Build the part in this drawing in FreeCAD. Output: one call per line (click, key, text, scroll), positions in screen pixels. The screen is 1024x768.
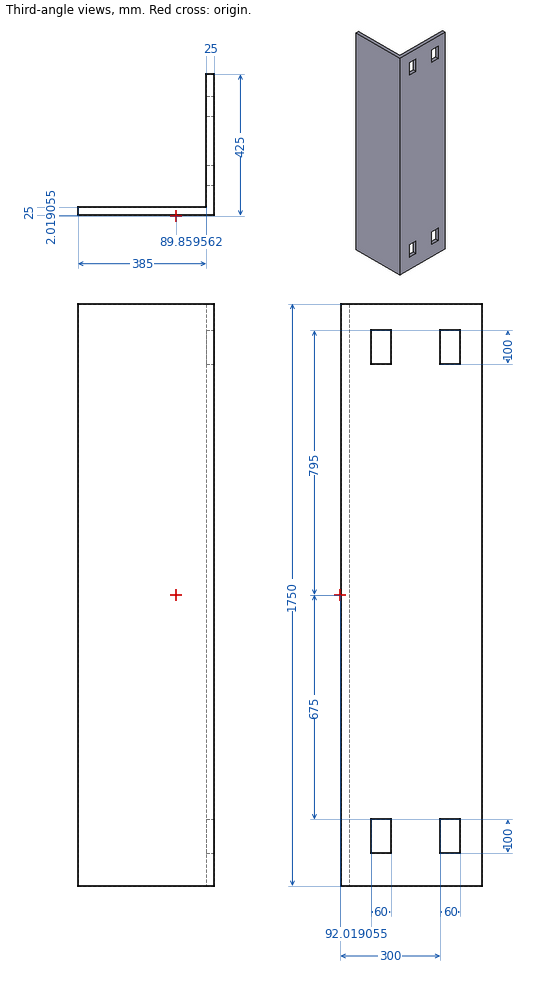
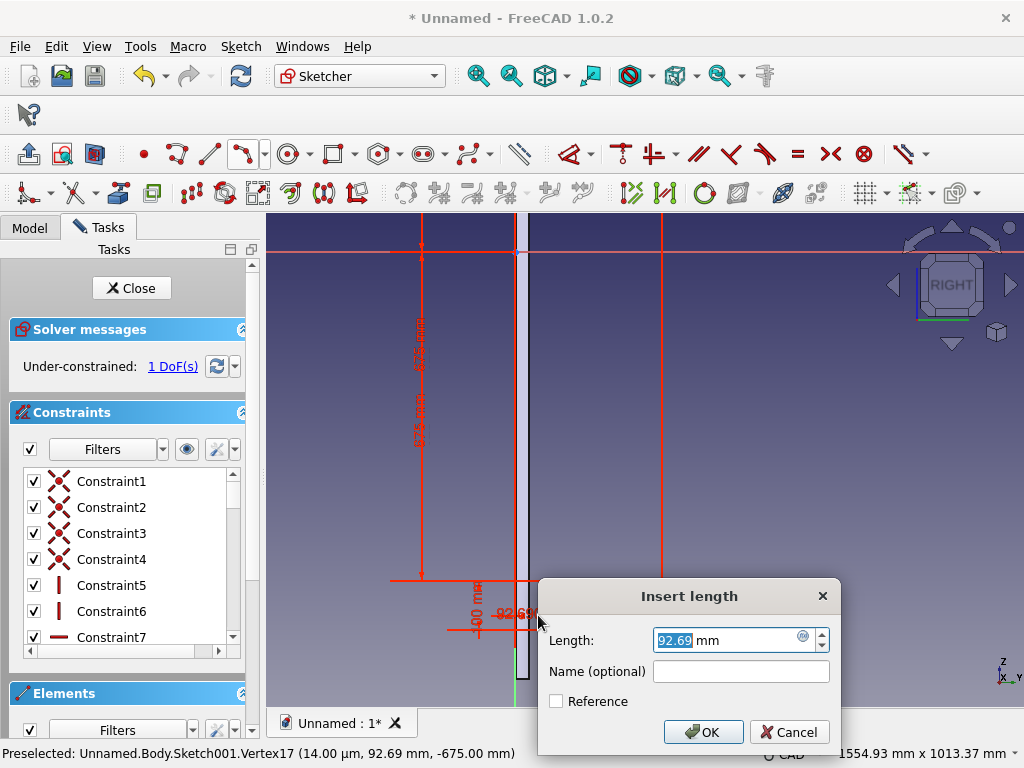
text(92.019055)
key(Return)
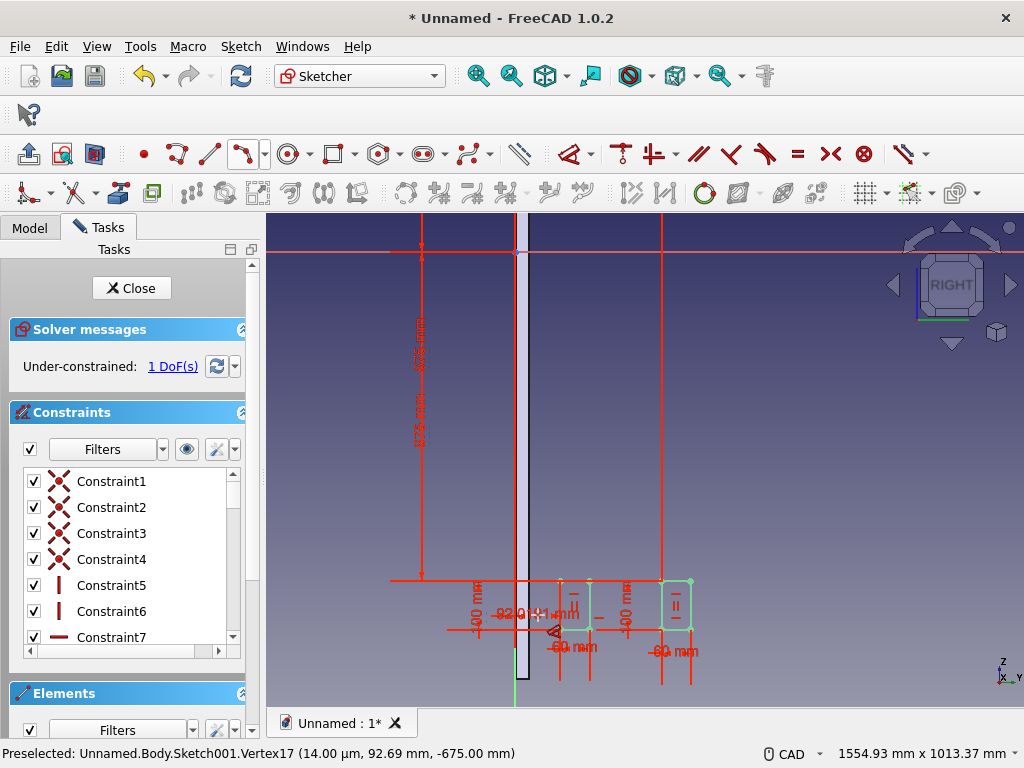
scroll(561, 584, down, 5)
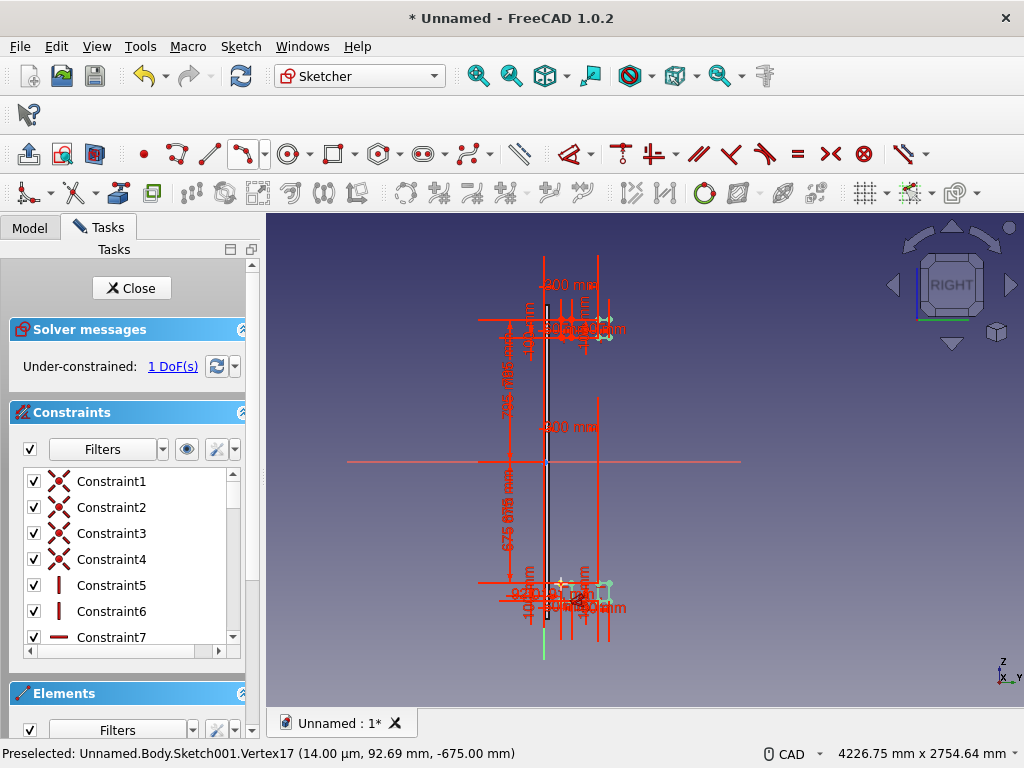
scroll(561, 320, up, 5)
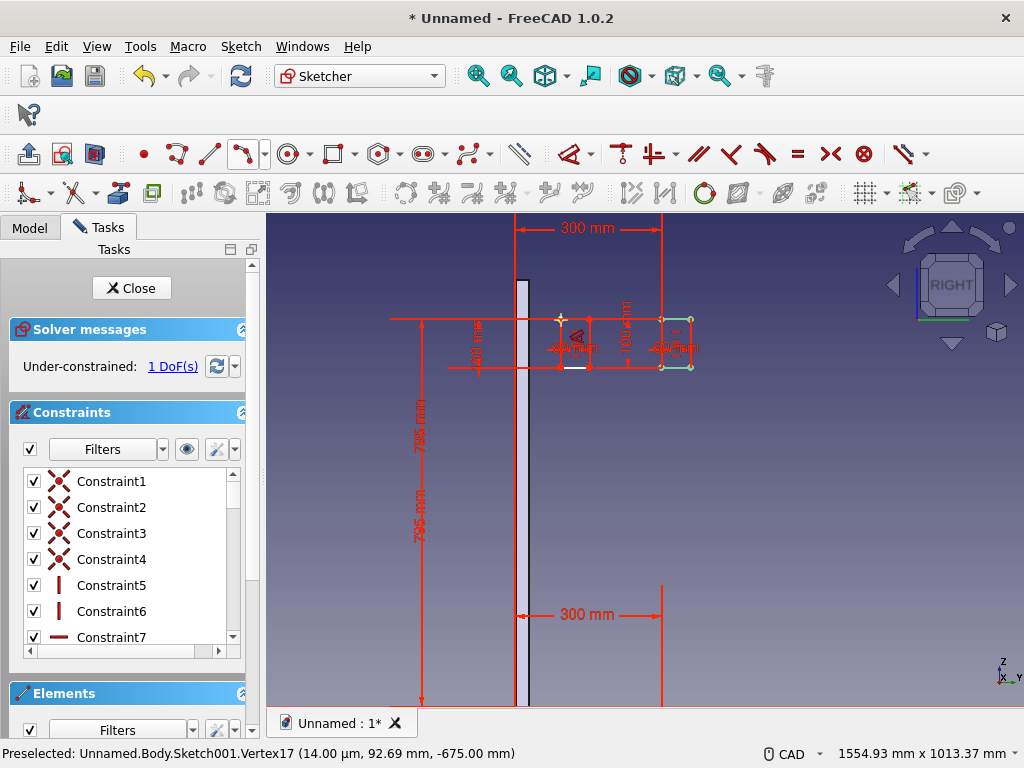
click(561, 319)
click(538, 285)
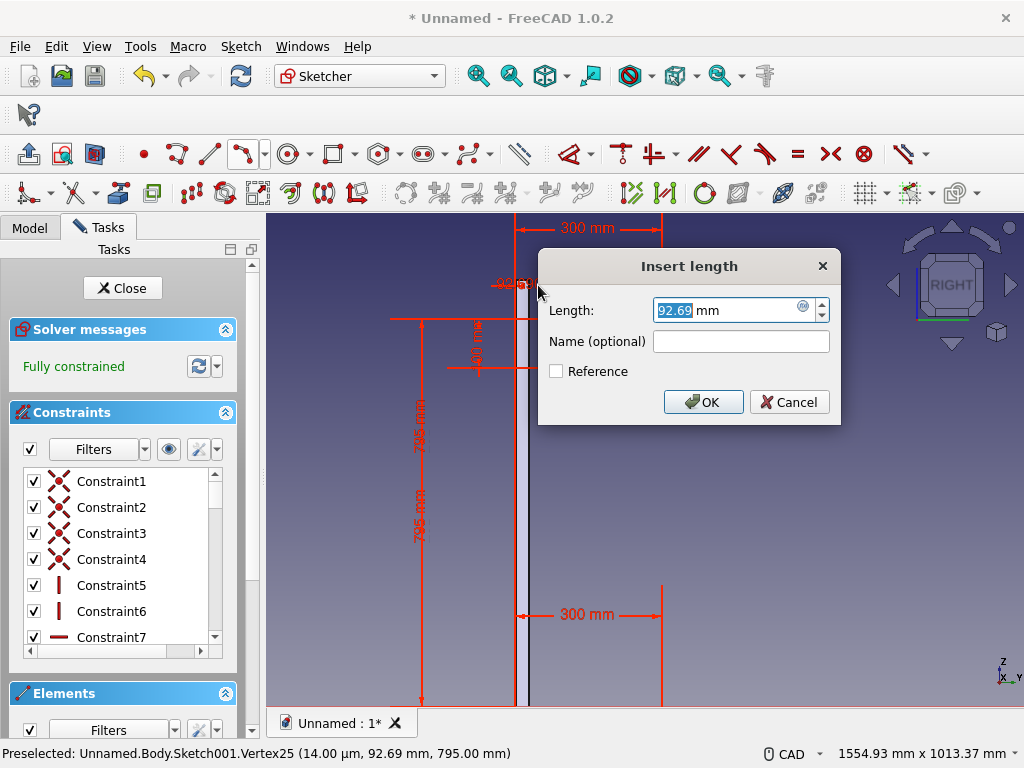
text(92.019055)
key(Return)
key(Escape)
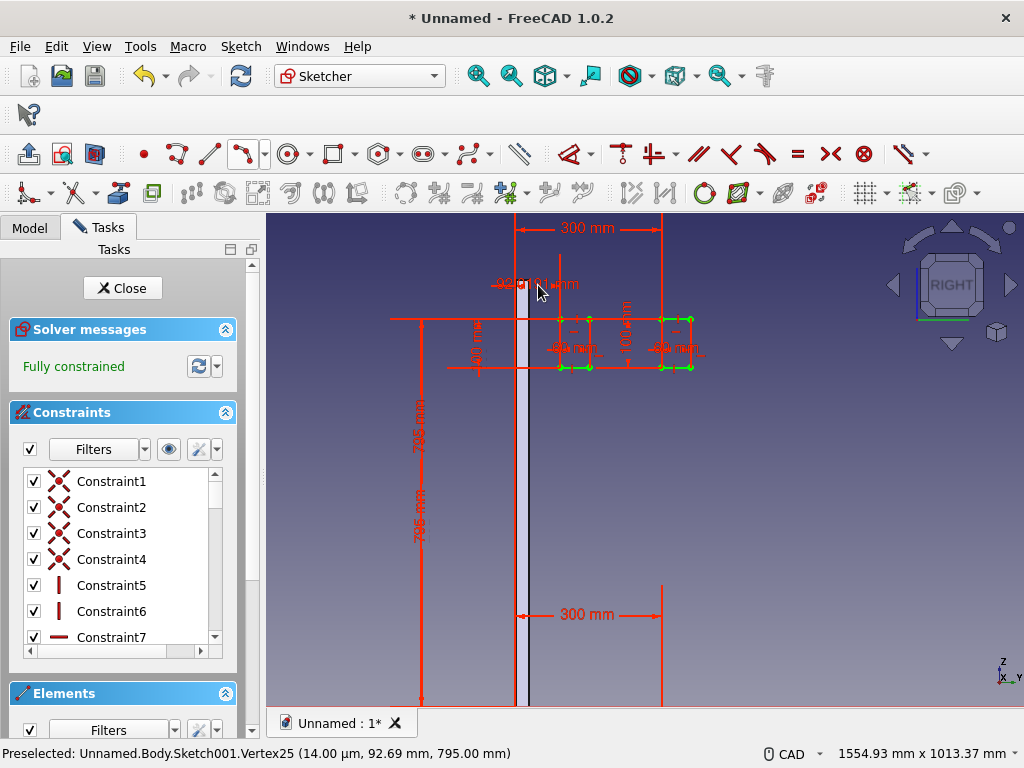
click(123, 288)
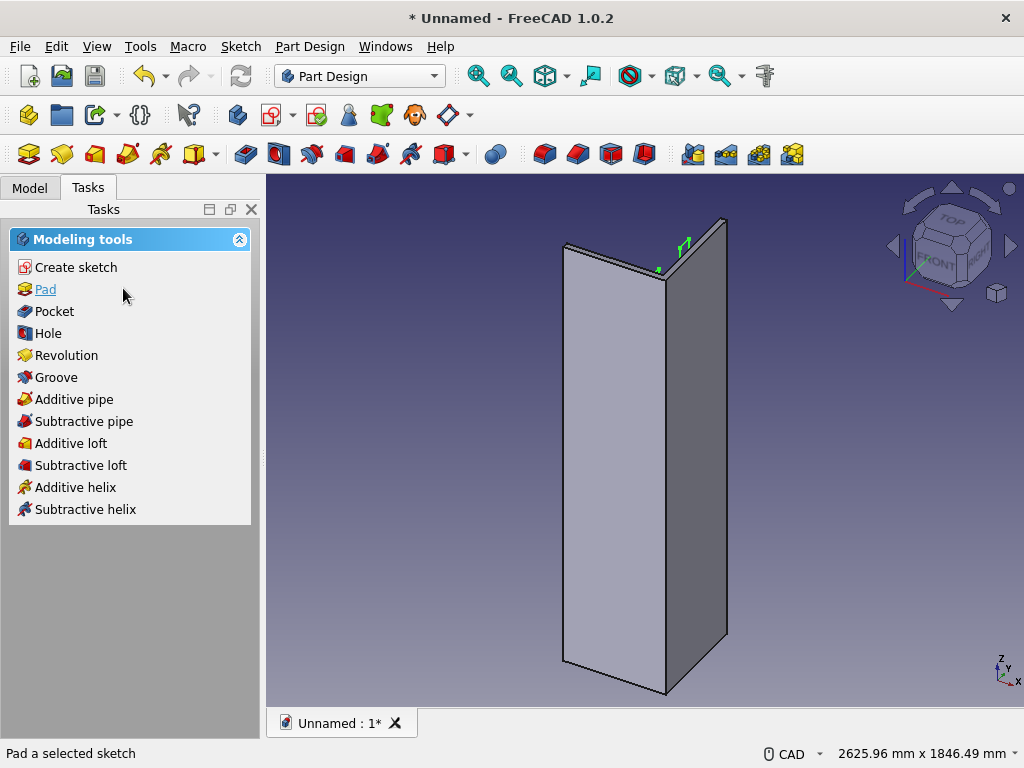
click(246, 154)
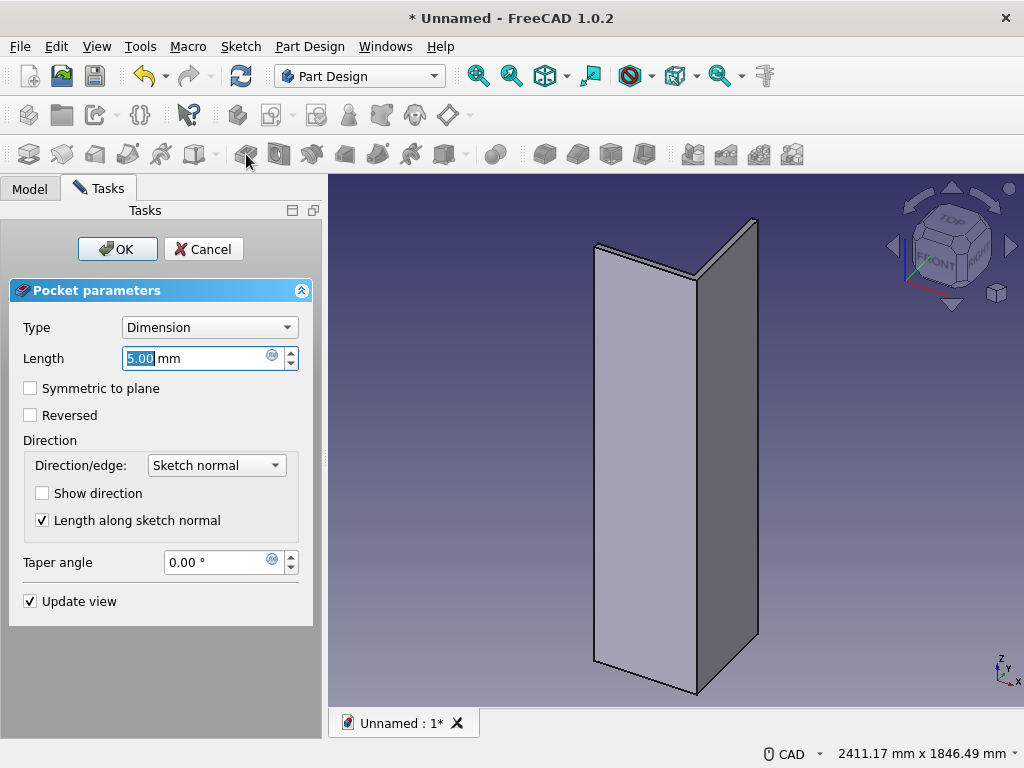
click(210, 328)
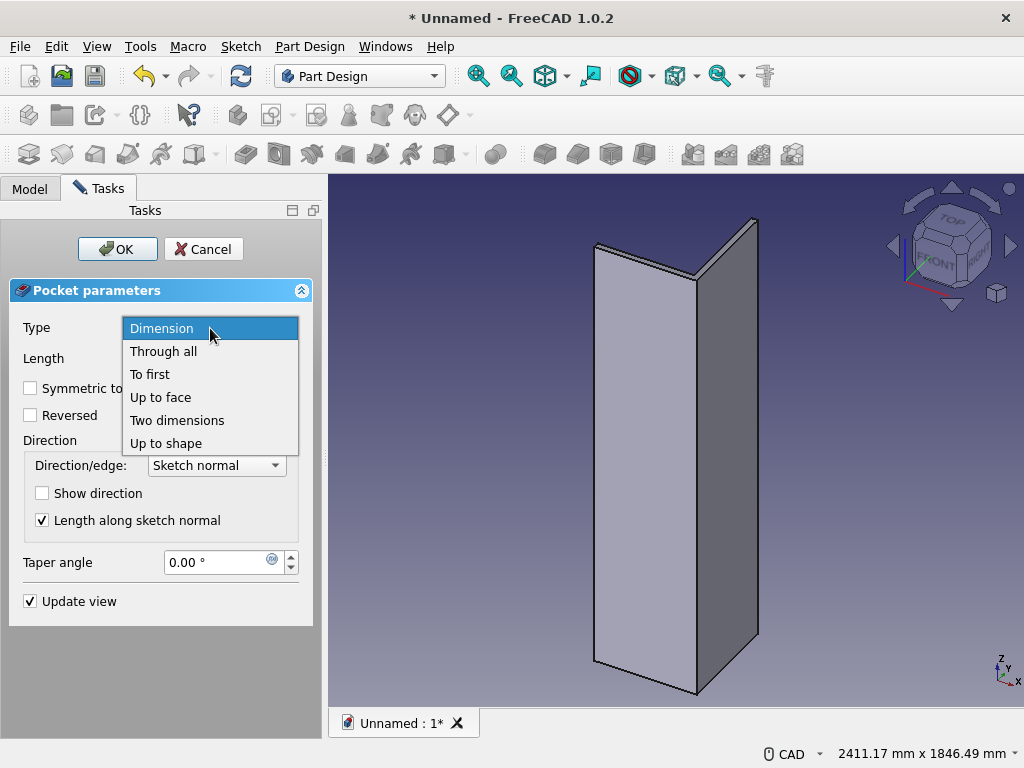
click(208, 352)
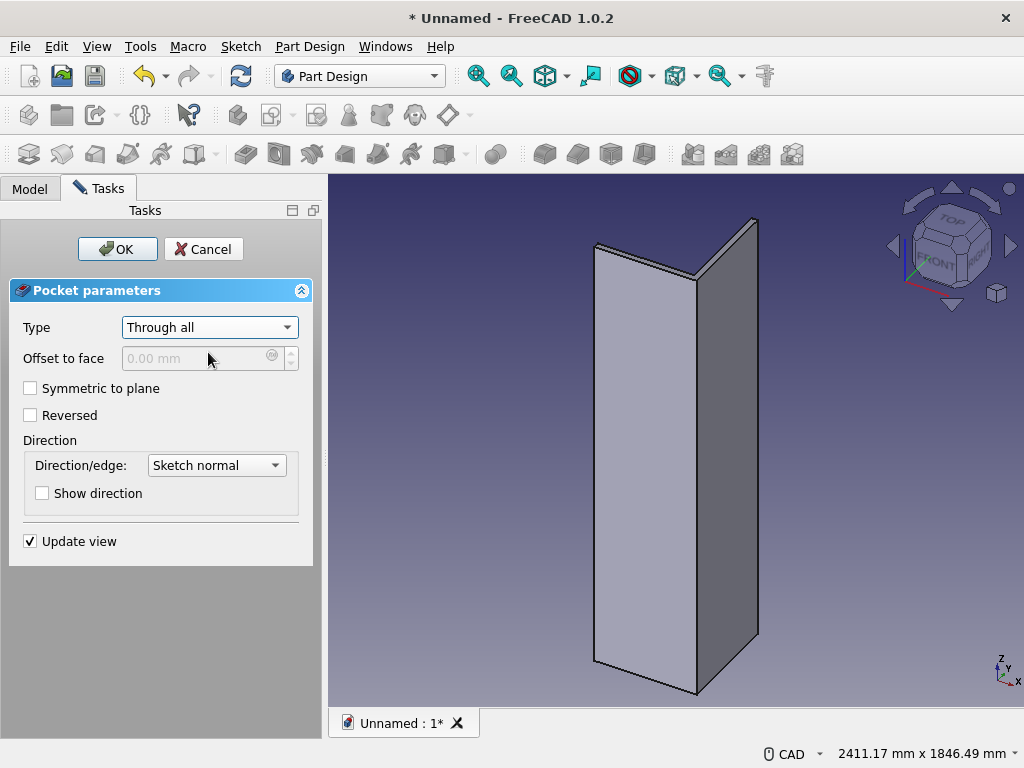
click(31, 415)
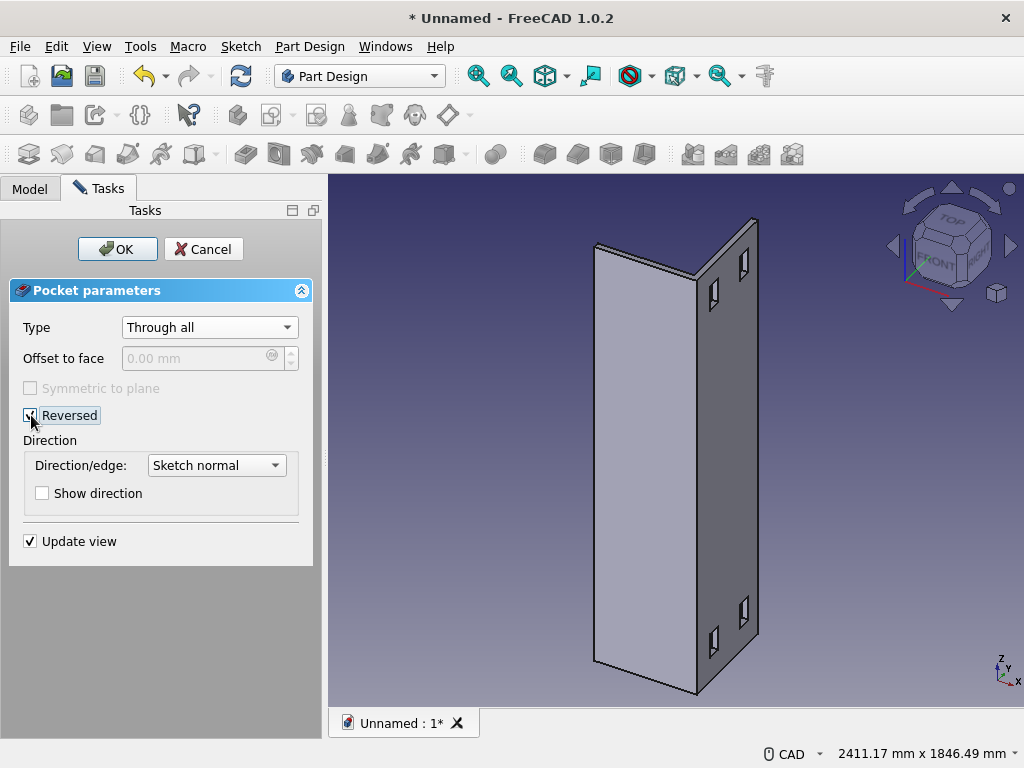
click(118, 249)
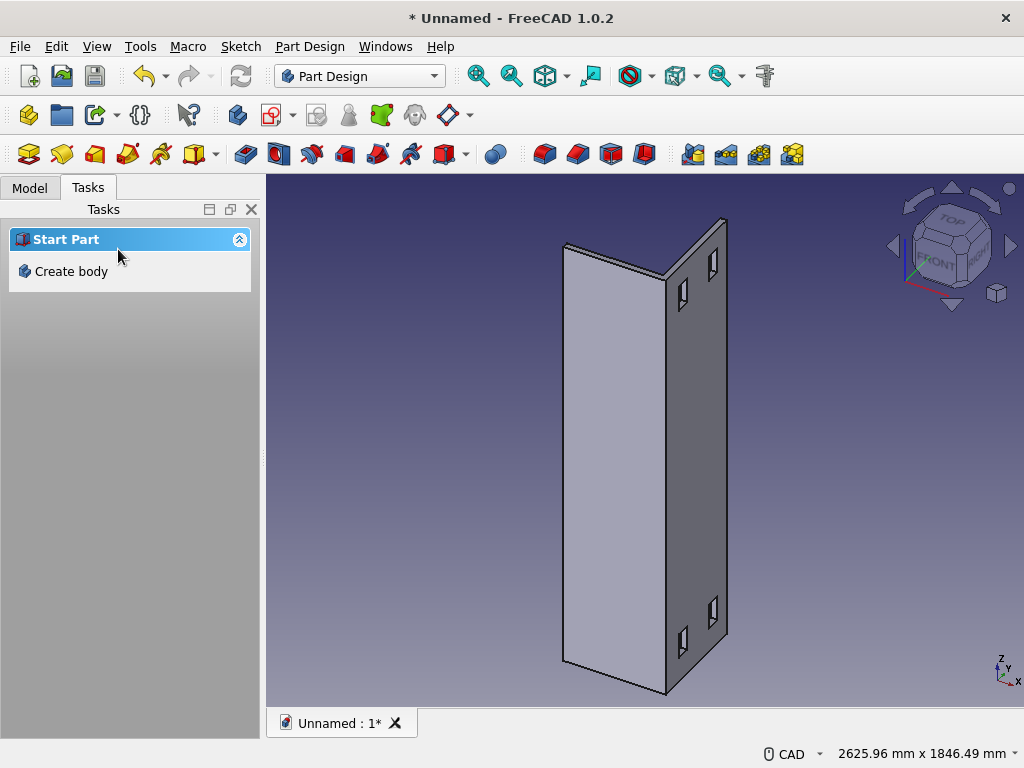
key(0)